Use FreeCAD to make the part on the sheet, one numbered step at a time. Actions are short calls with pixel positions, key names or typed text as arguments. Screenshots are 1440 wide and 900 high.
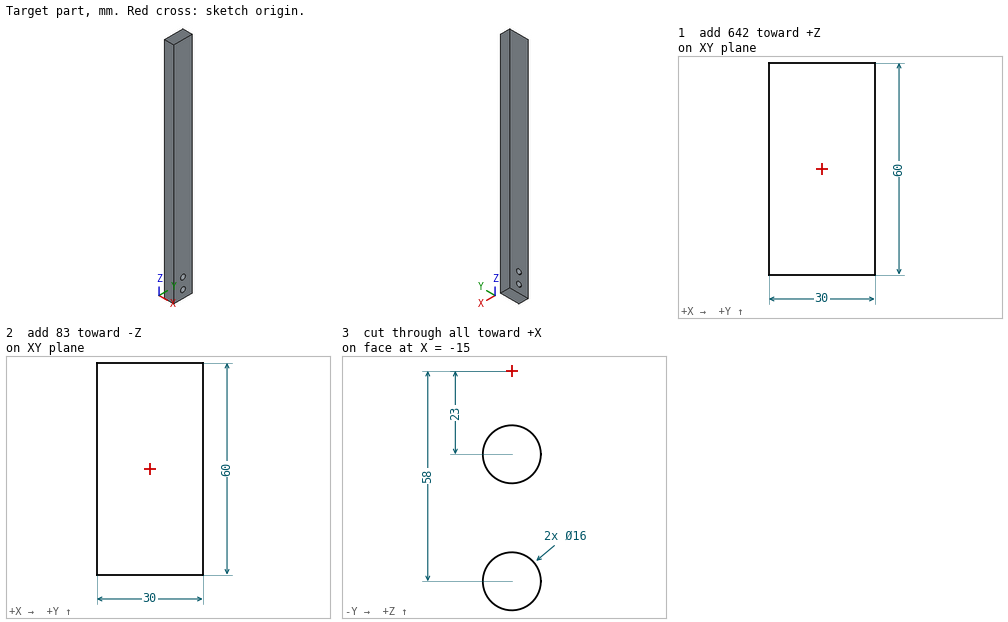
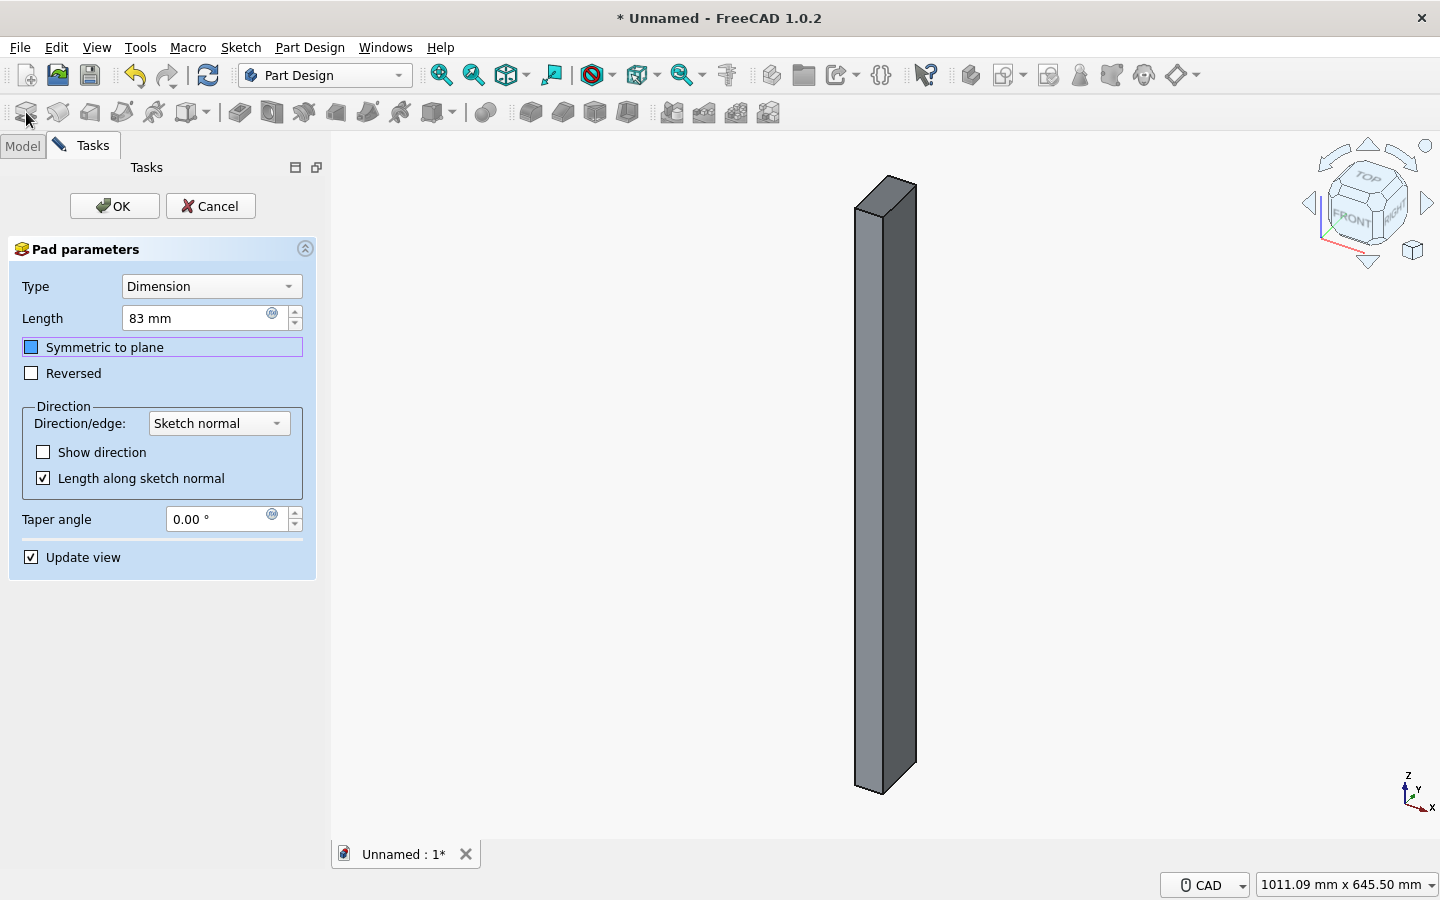
click(30, 373)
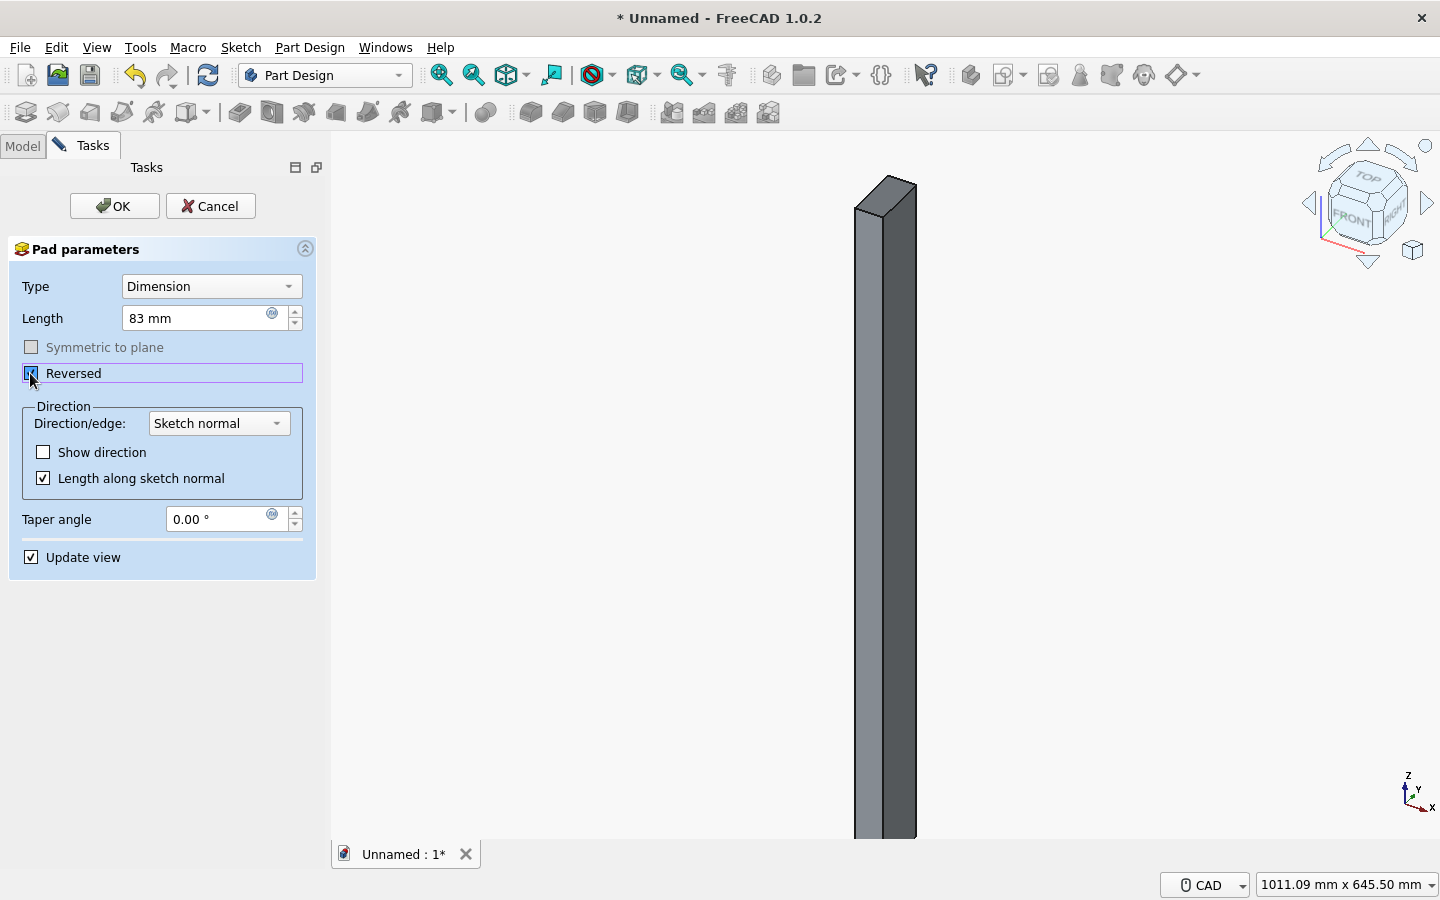
click(115, 206)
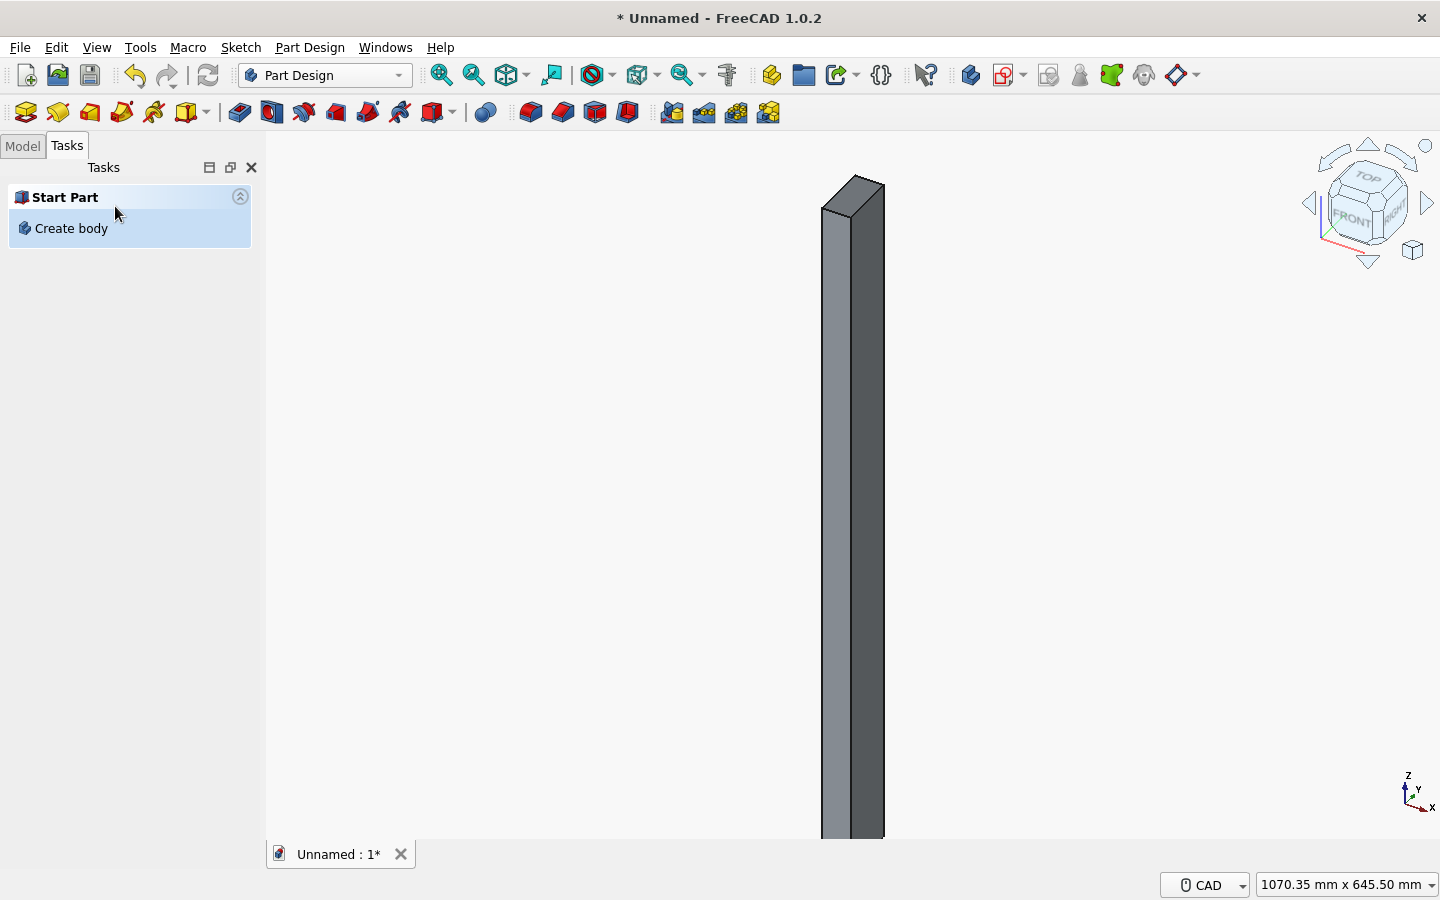
click(442, 76)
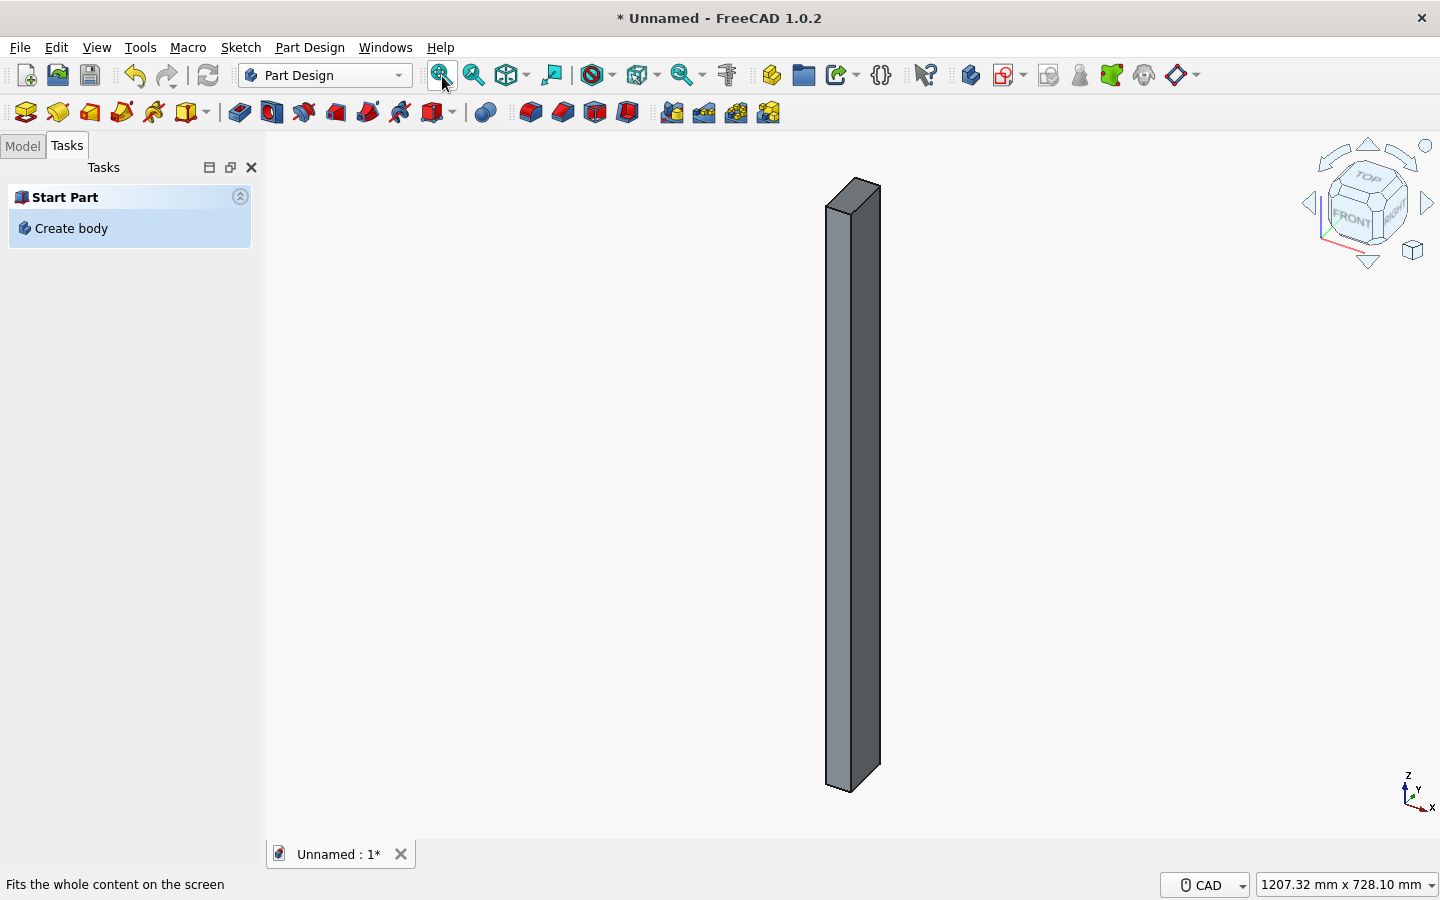
key(6)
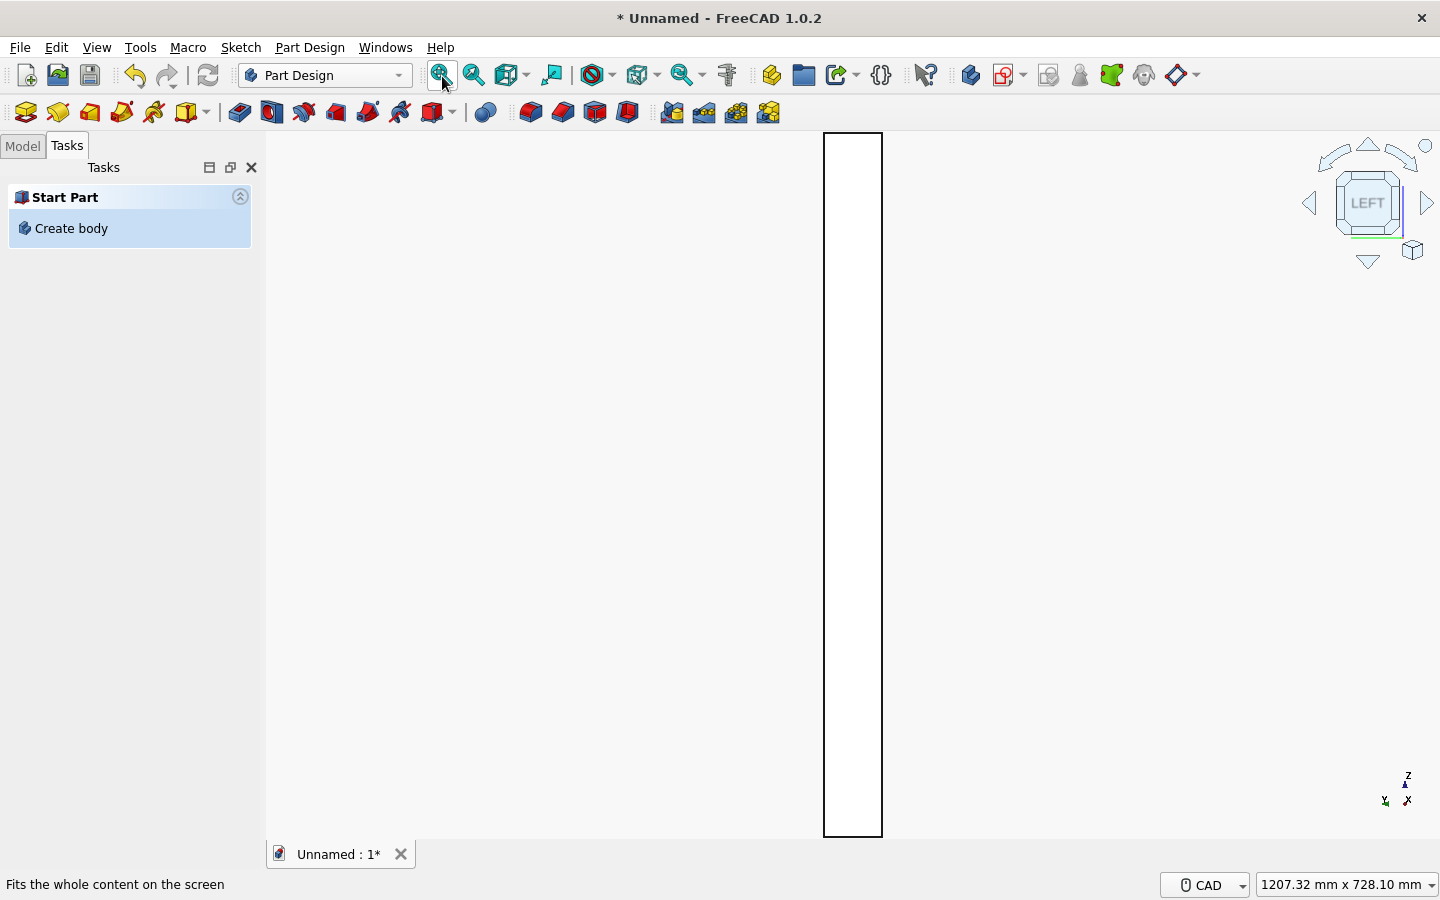
click(853, 182)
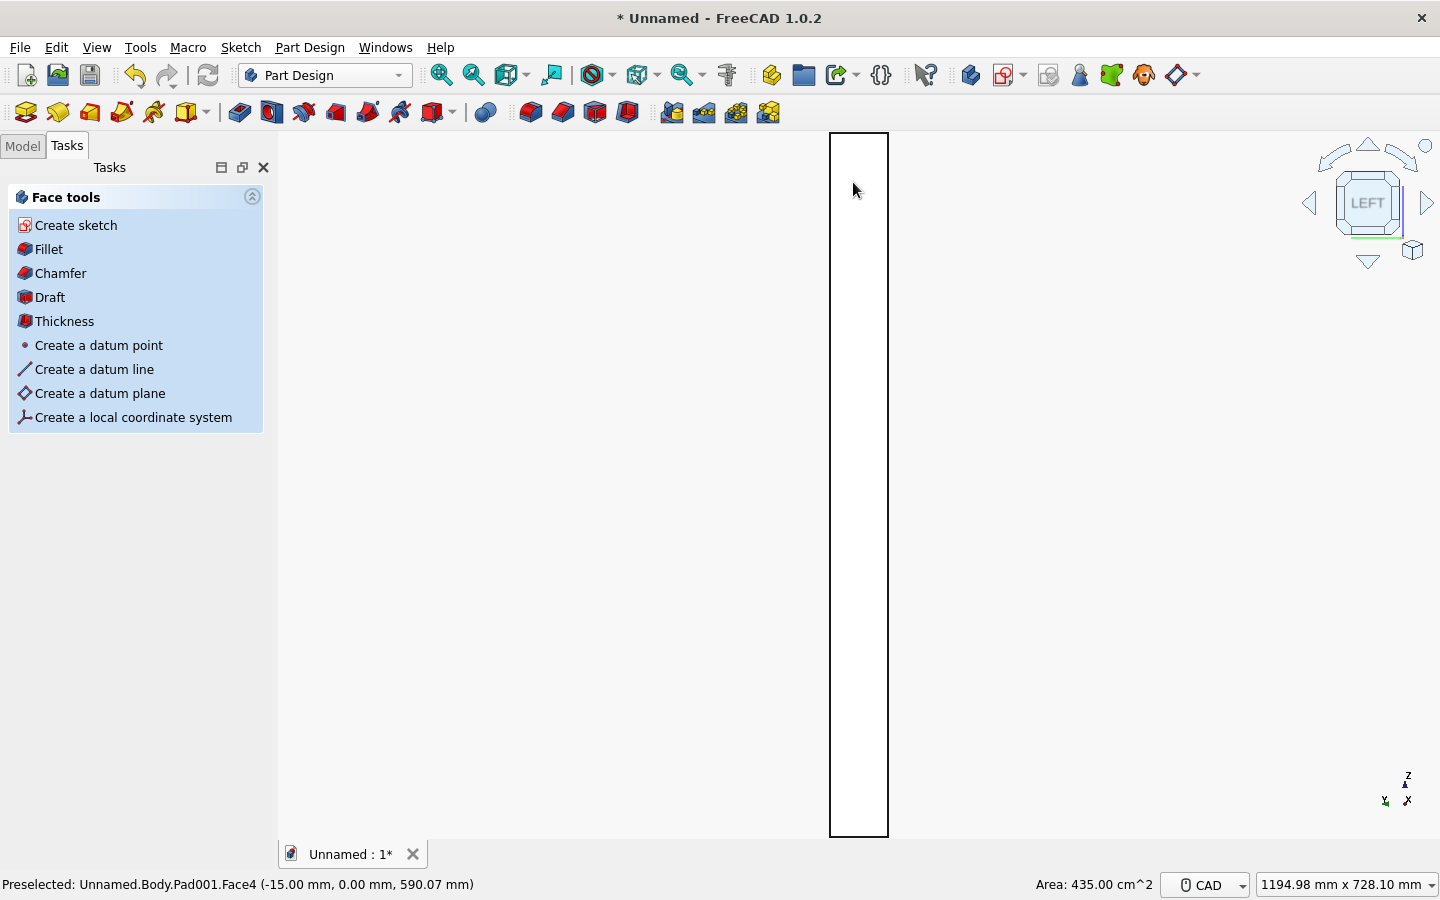
click(1004, 76)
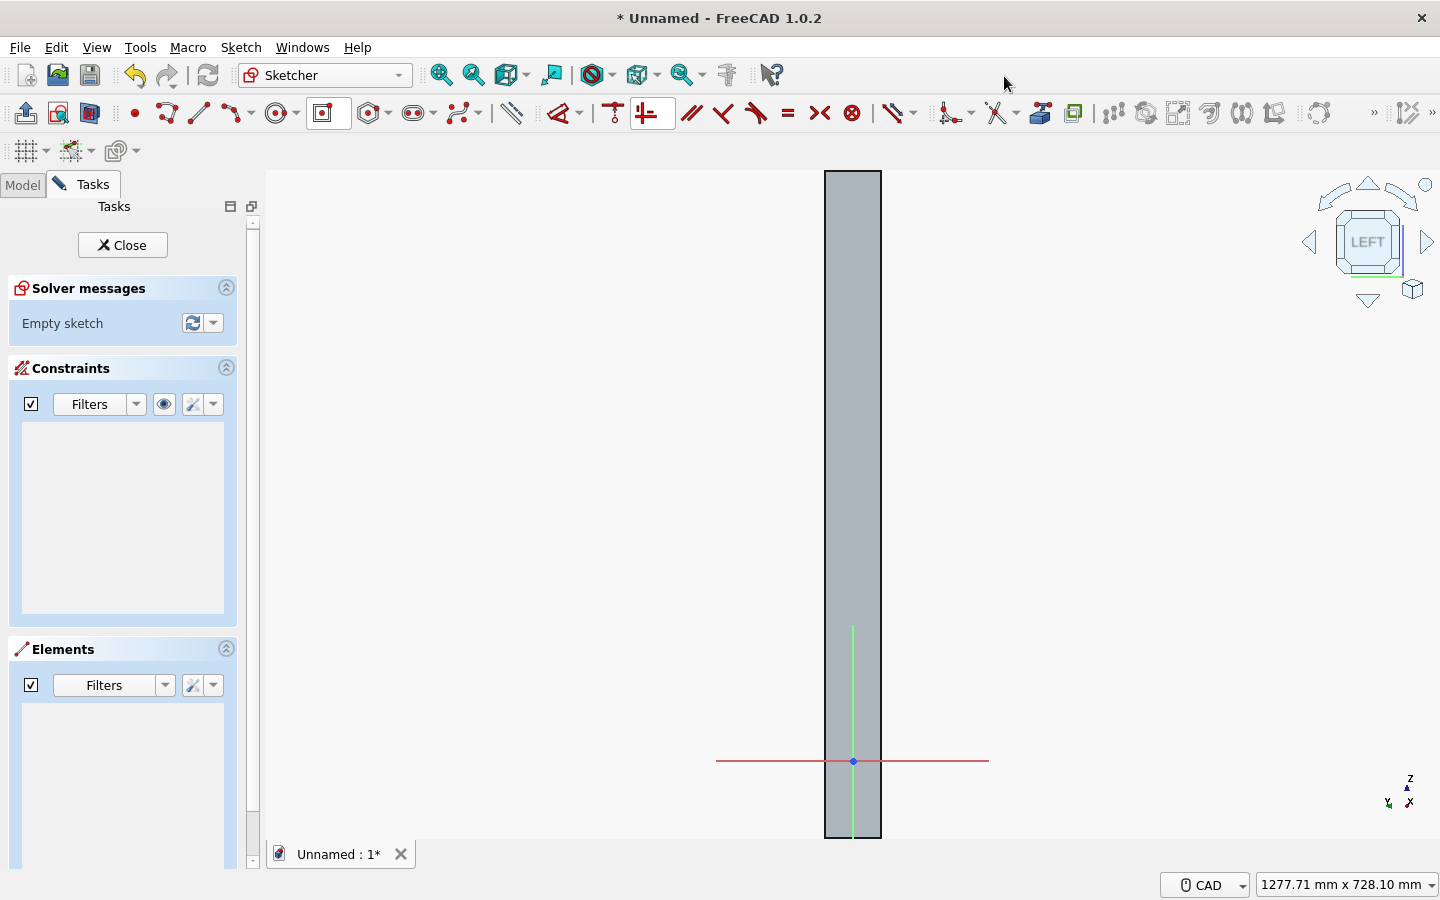
scroll(784, 504, down, 5)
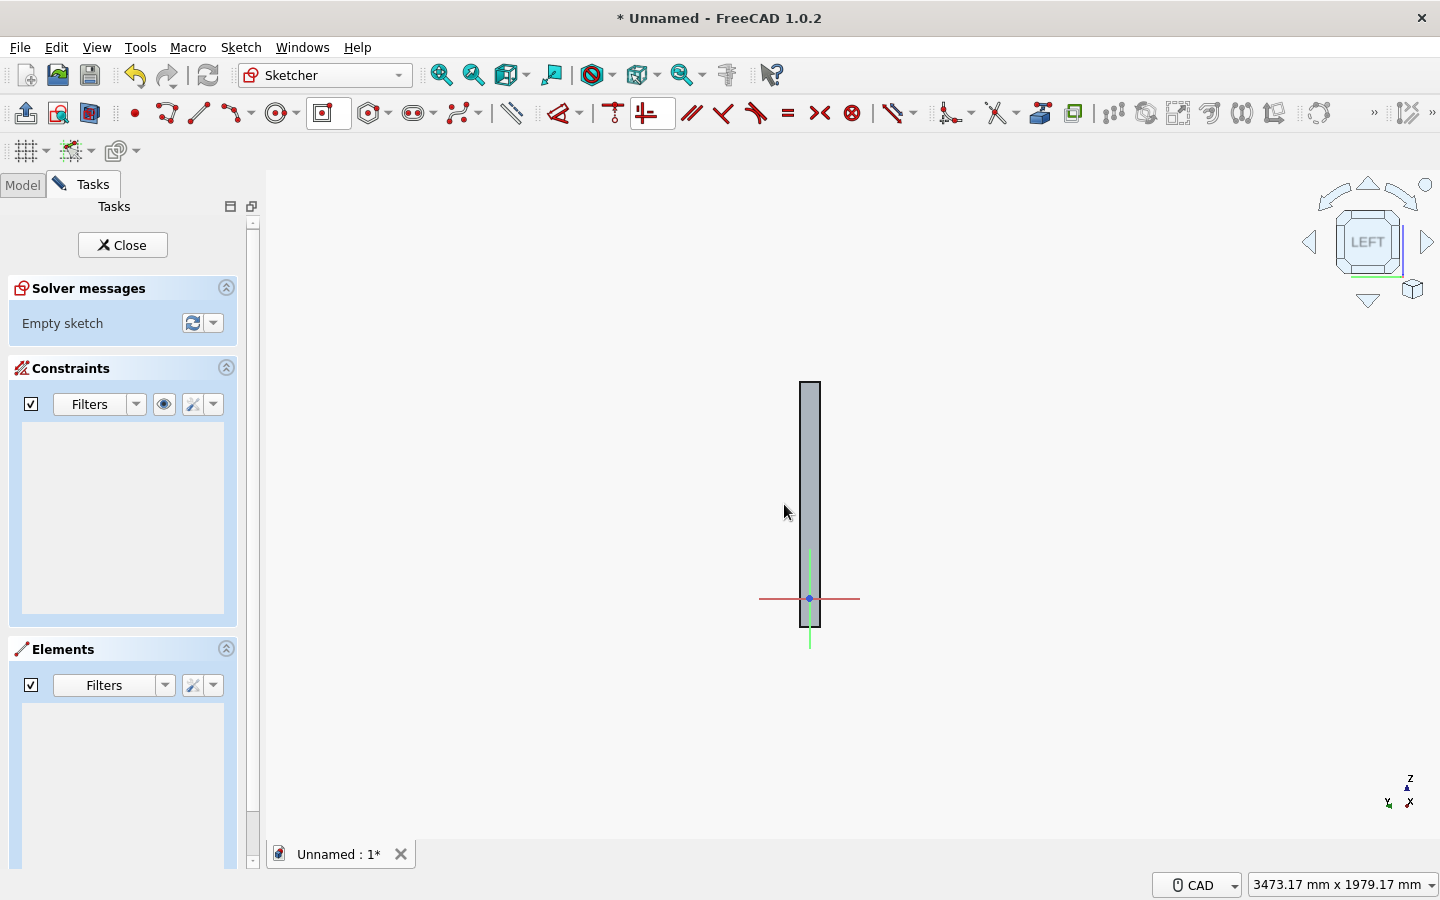
scroll(811, 616, up, 15)